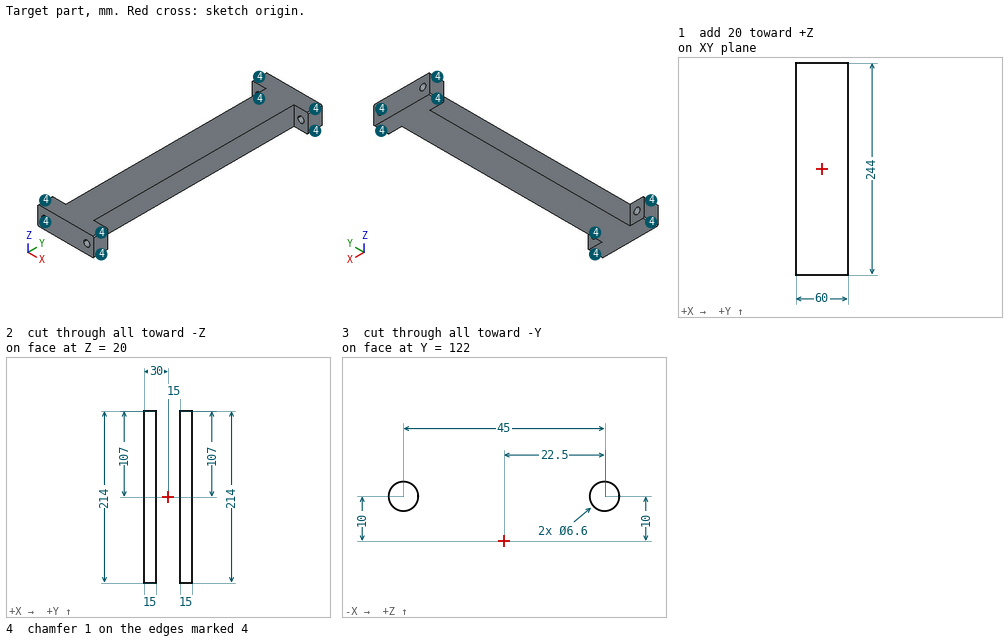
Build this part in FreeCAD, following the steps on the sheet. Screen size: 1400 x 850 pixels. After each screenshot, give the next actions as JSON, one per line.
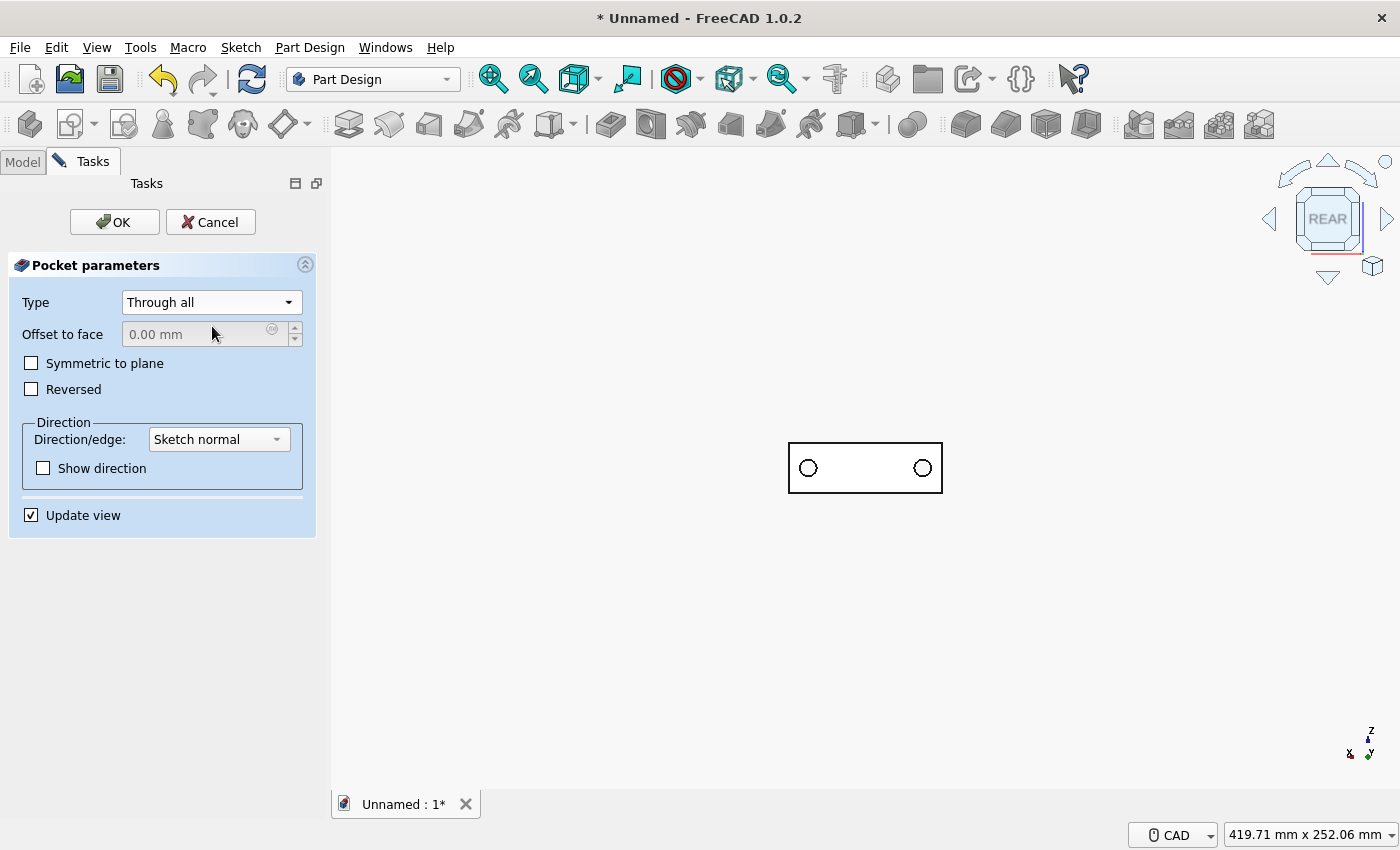
{"action": "left_click", "coordinate": [115, 222]}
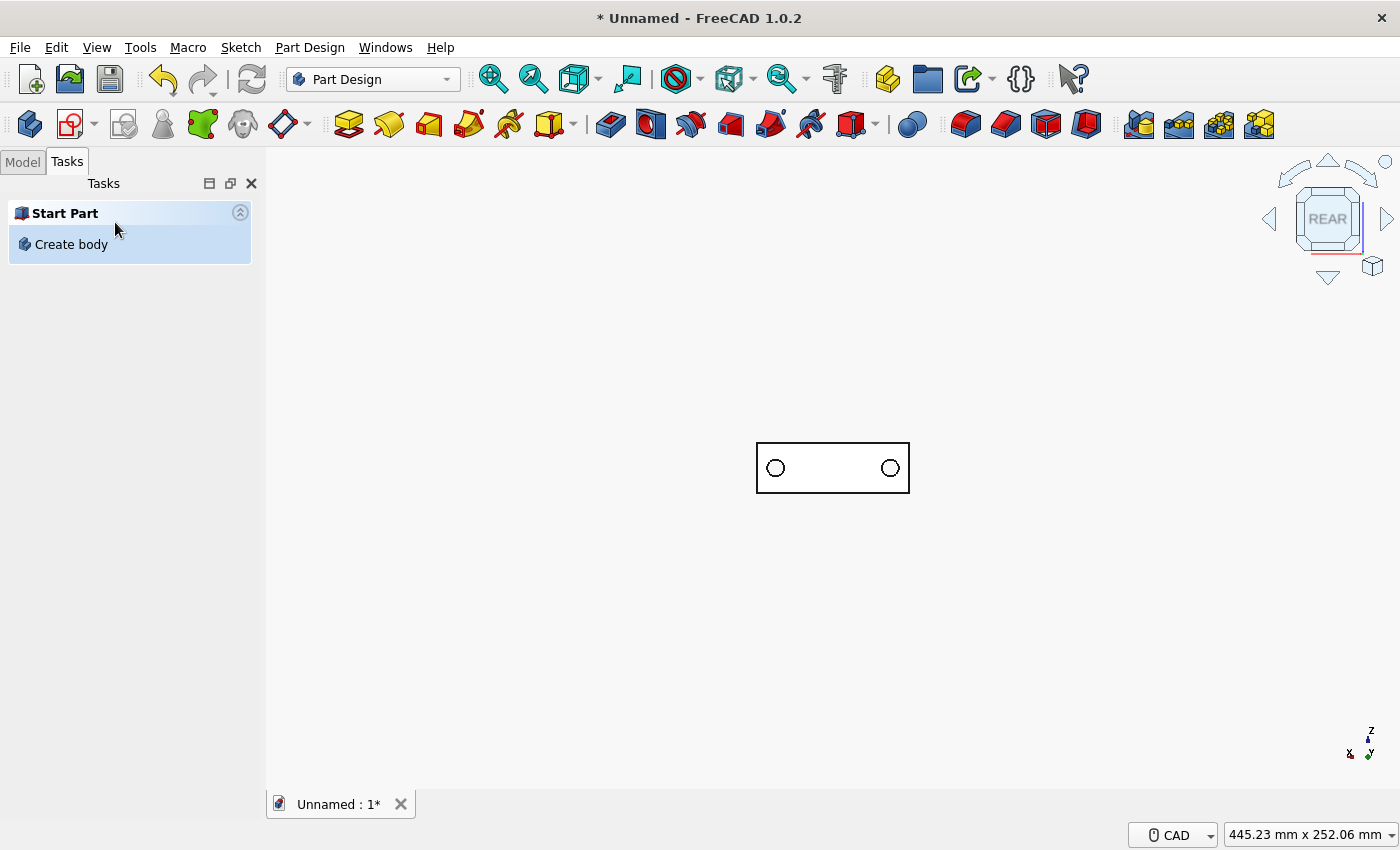
{"action": "left_click", "coordinate": [494, 80]}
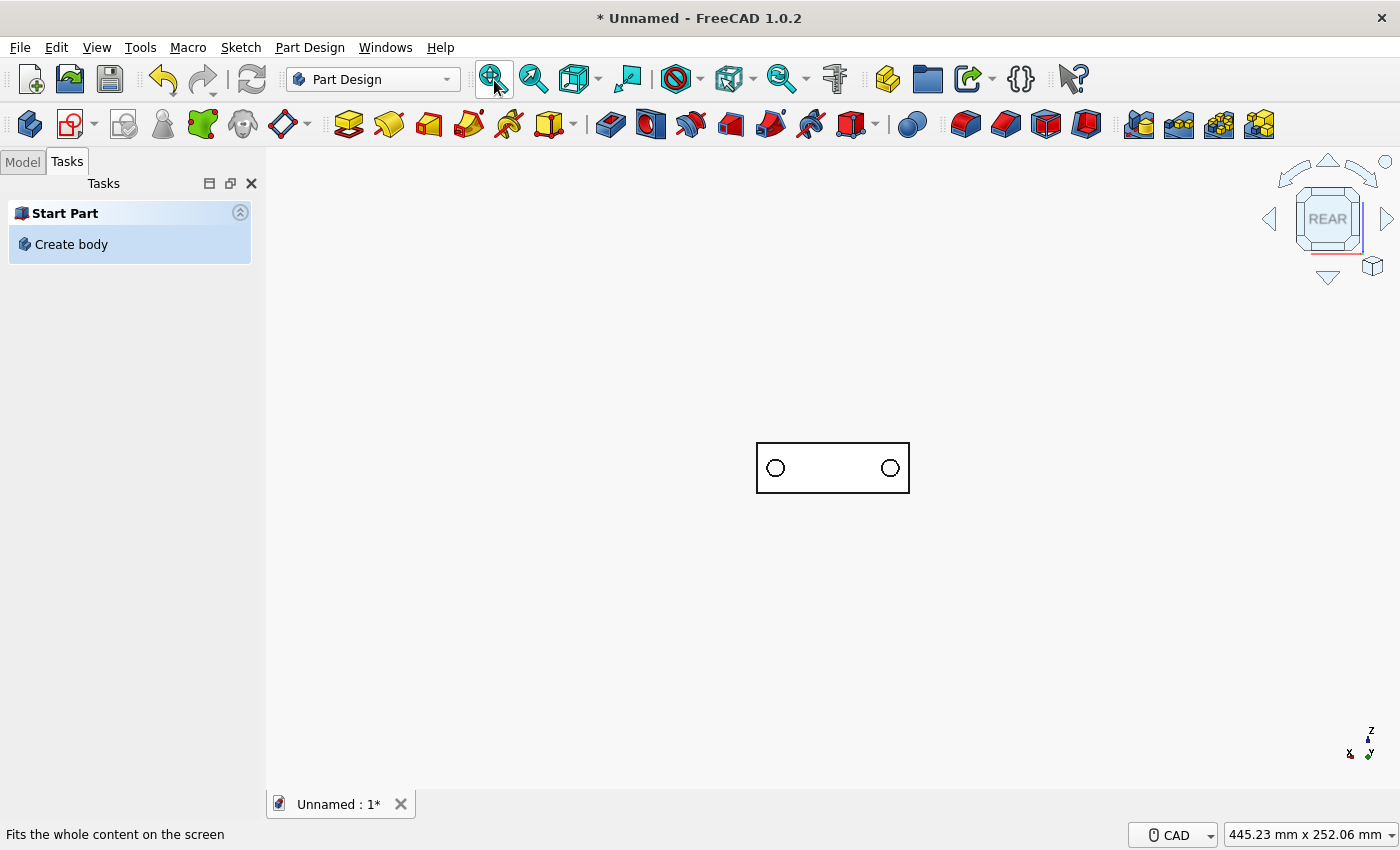
{"action": "key", "text": "0"}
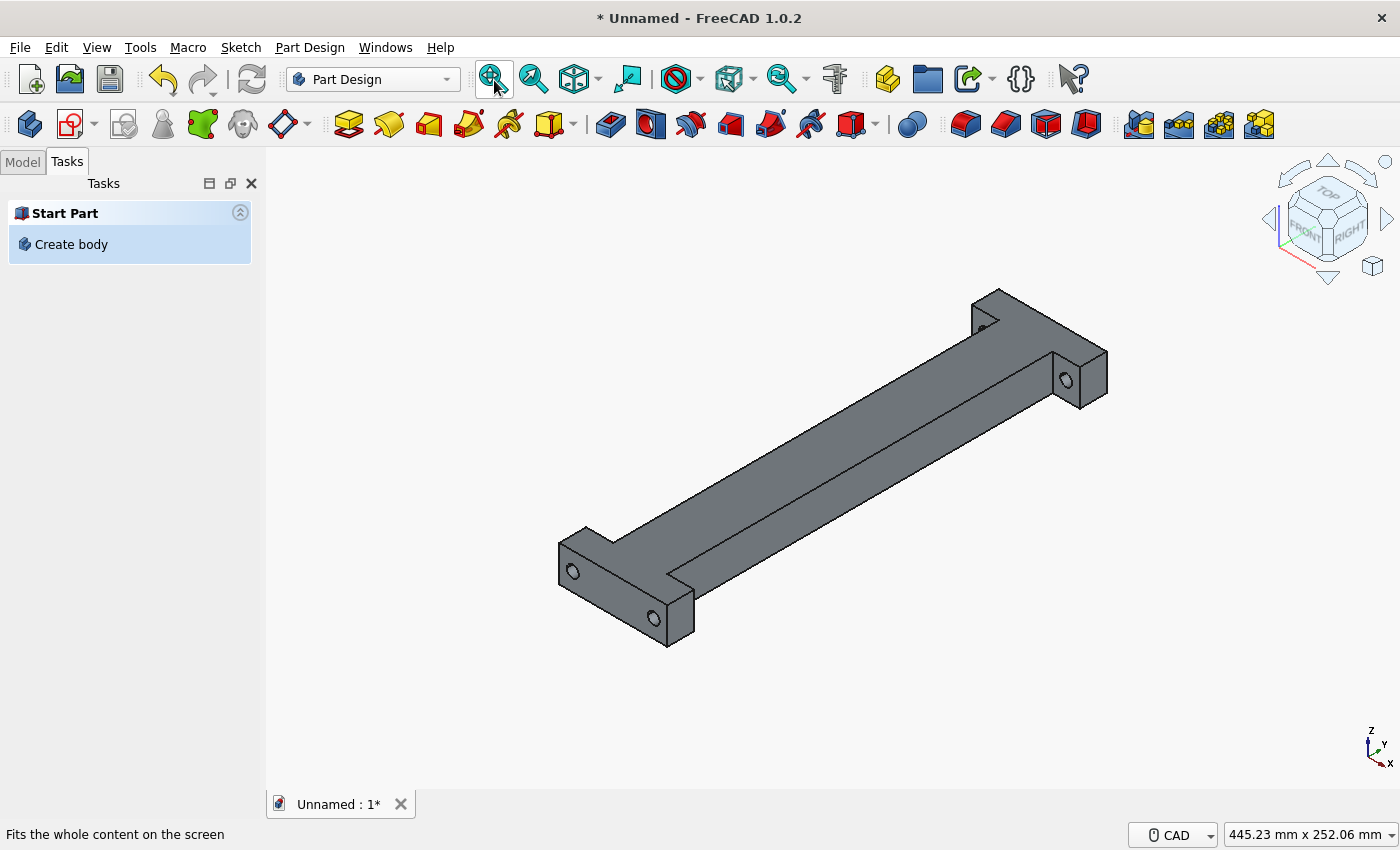
{"action": "left_click", "coordinate": [1093, 358]}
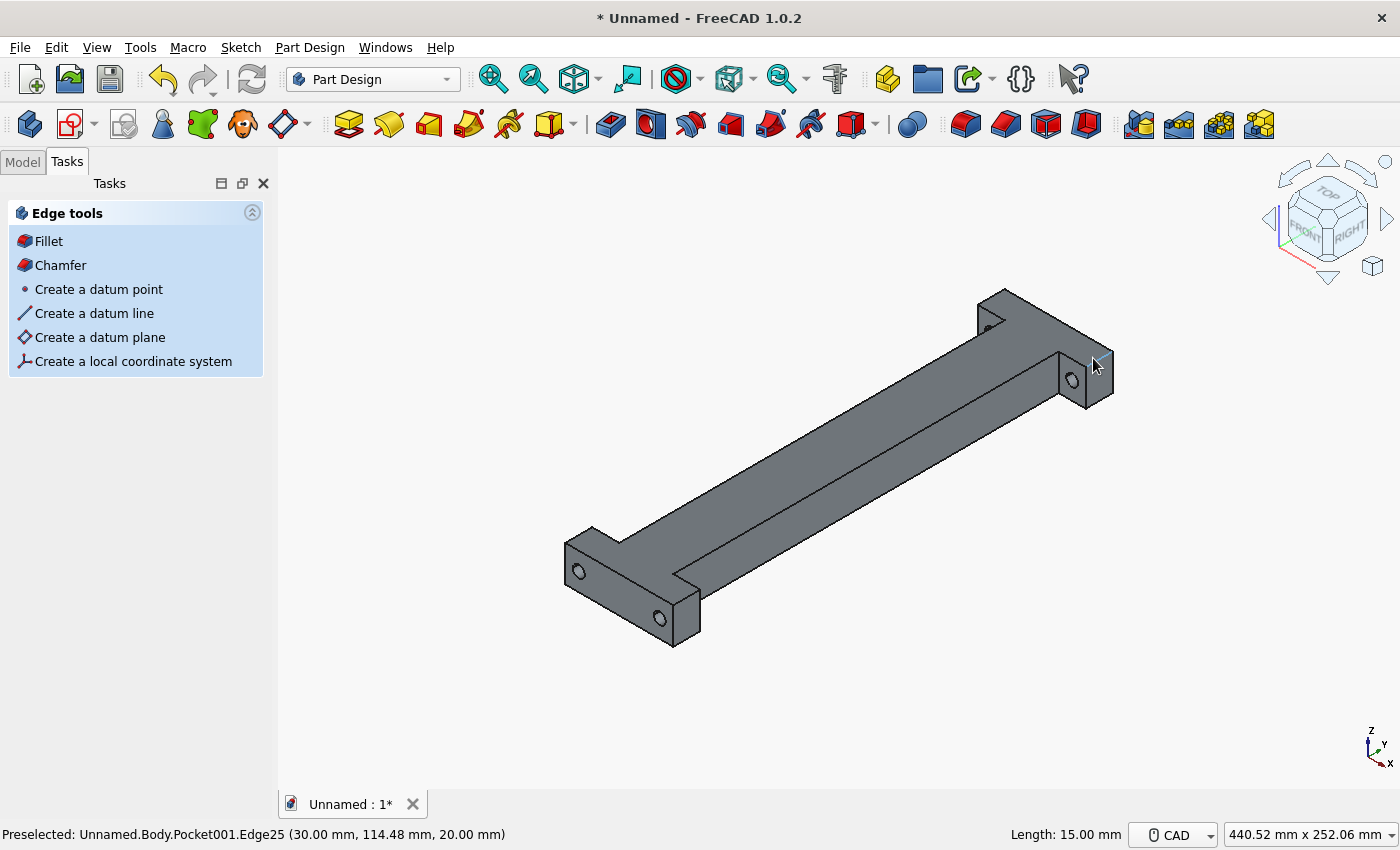
{"action": "left_click", "coordinate": [687, 596], "text": "ctrl"}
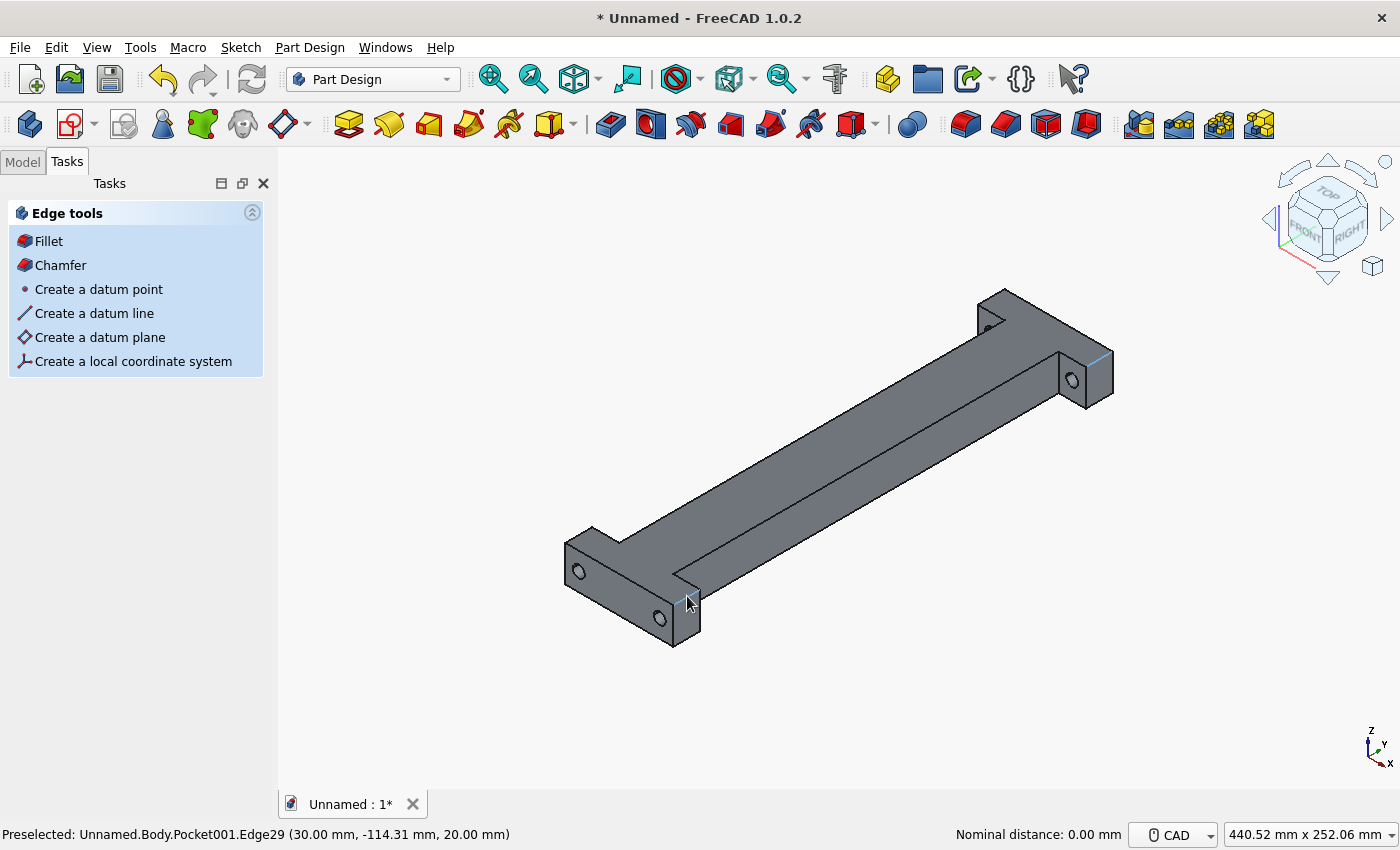
{"action": "key", "text": "2"}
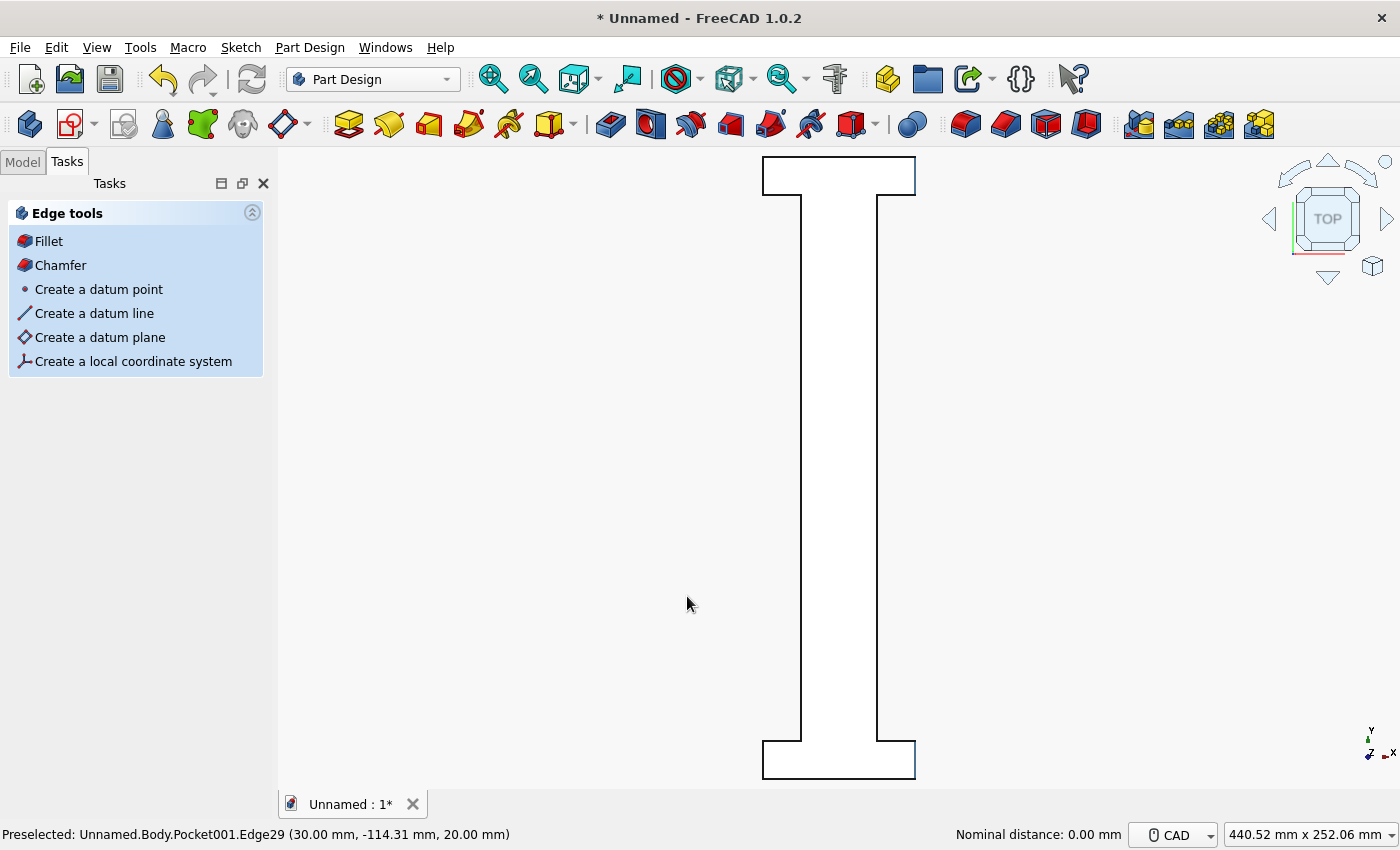
{"action": "left_click", "coordinate": [763, 179], "text": "ctrl"}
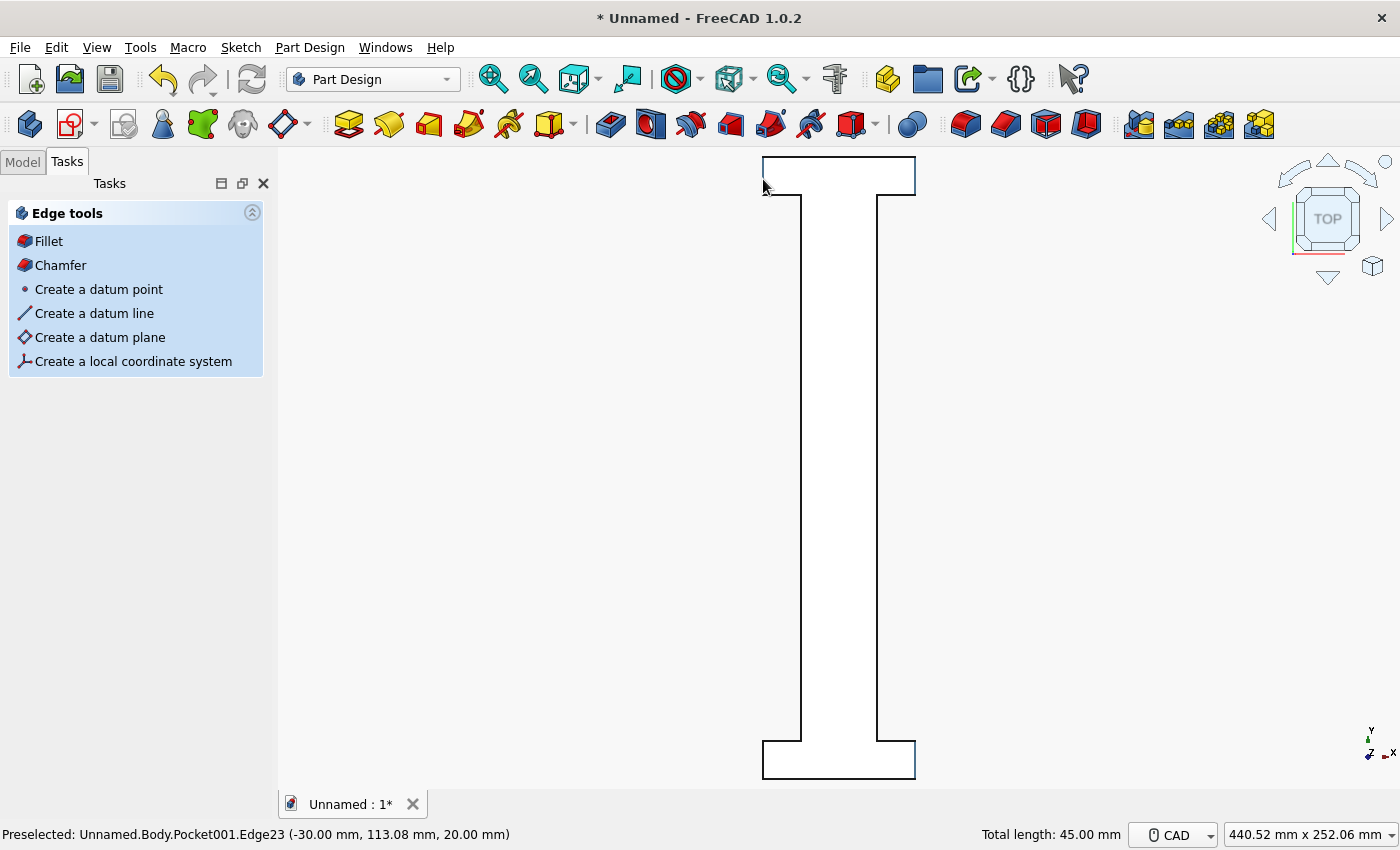
{"action": "left_click", "coordinate": [763, 759], "text": "ctrl"}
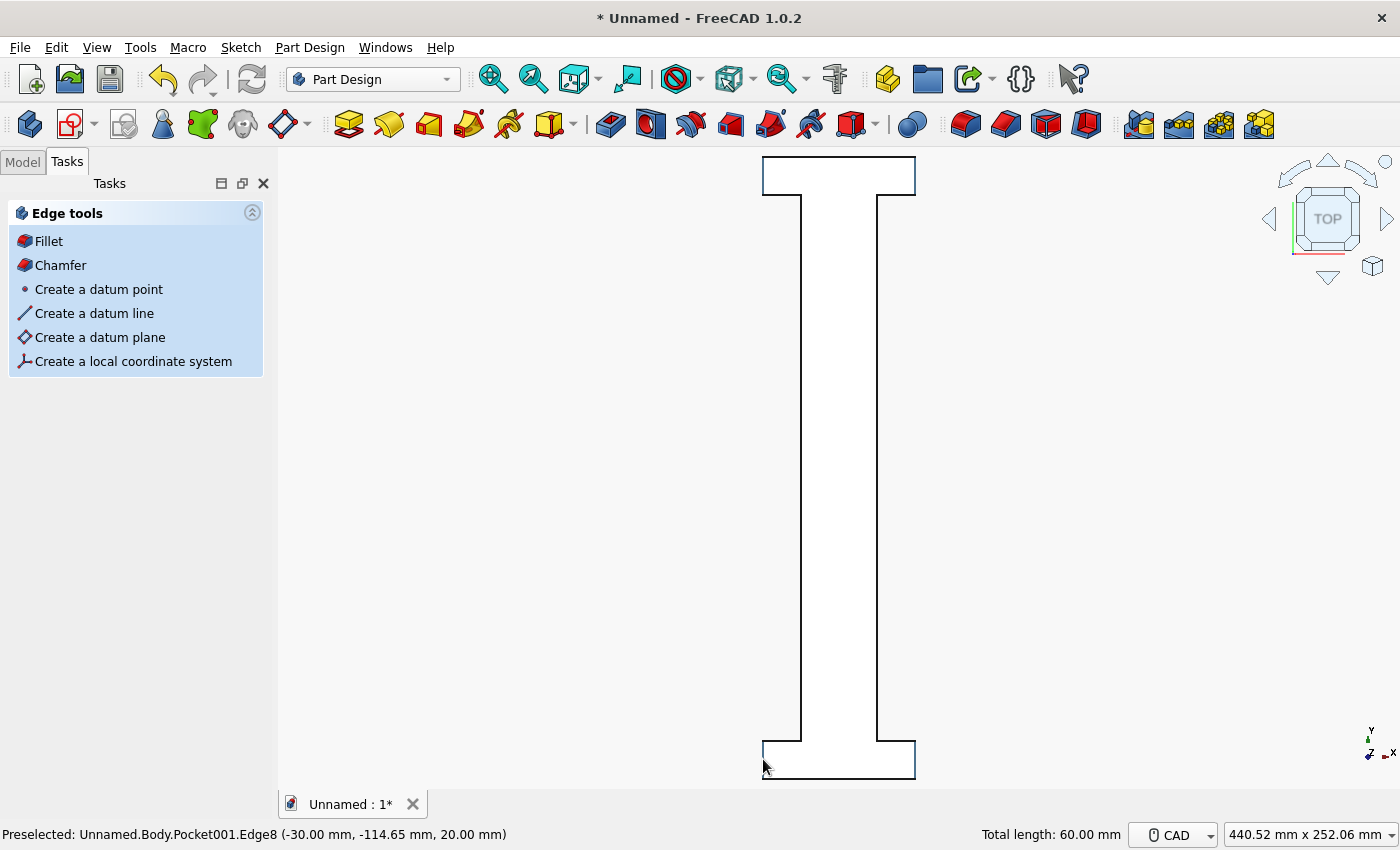
{"action": "key", "text": "1"}